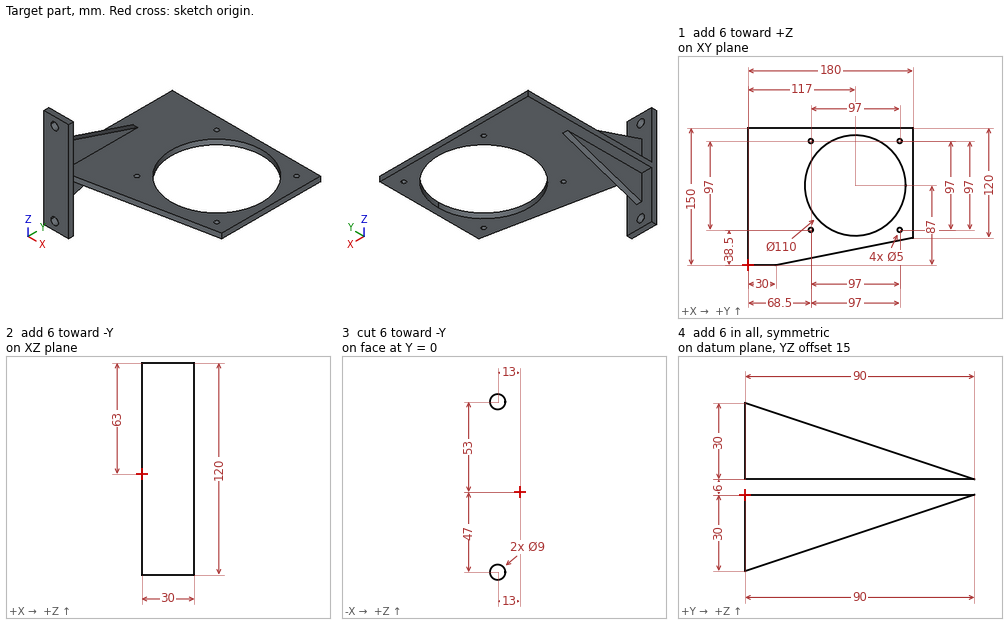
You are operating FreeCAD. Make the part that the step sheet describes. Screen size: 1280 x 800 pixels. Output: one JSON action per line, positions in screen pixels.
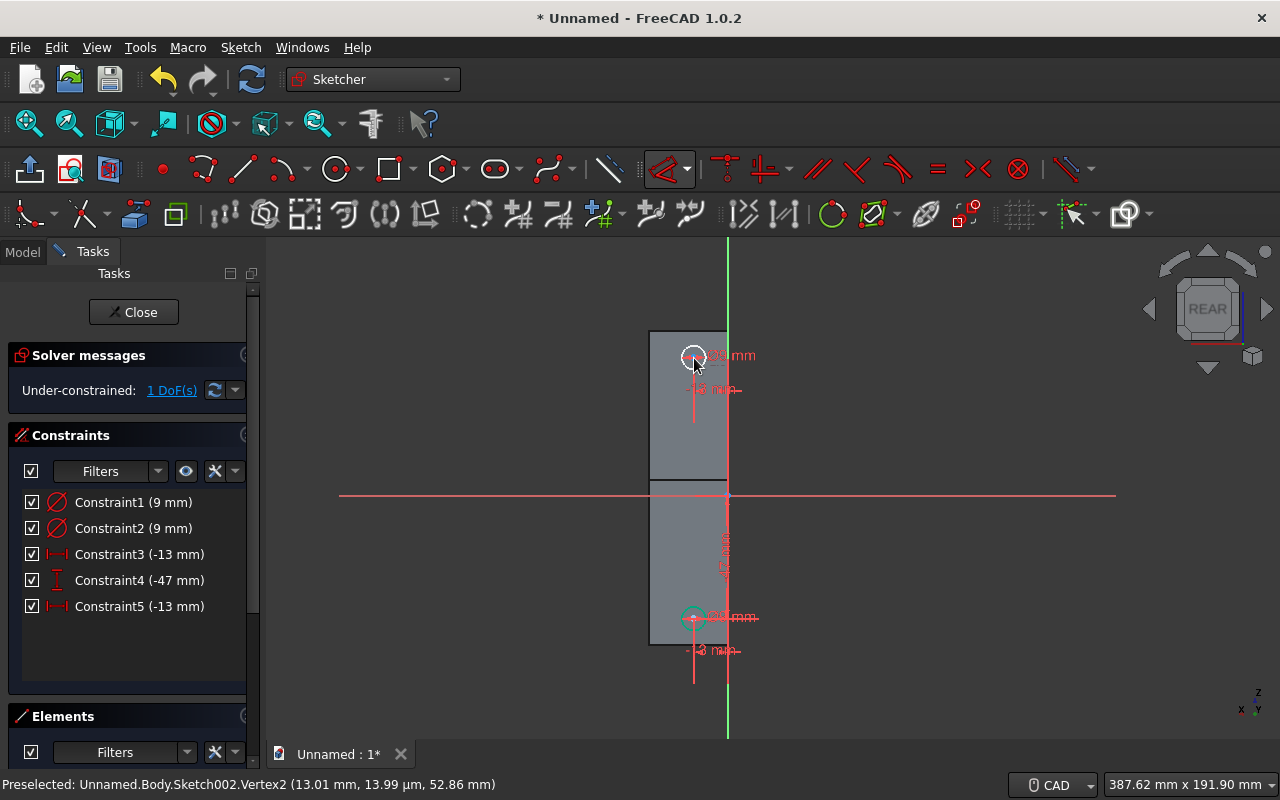
{"action": "left_click", "coordinate": [694, 358]}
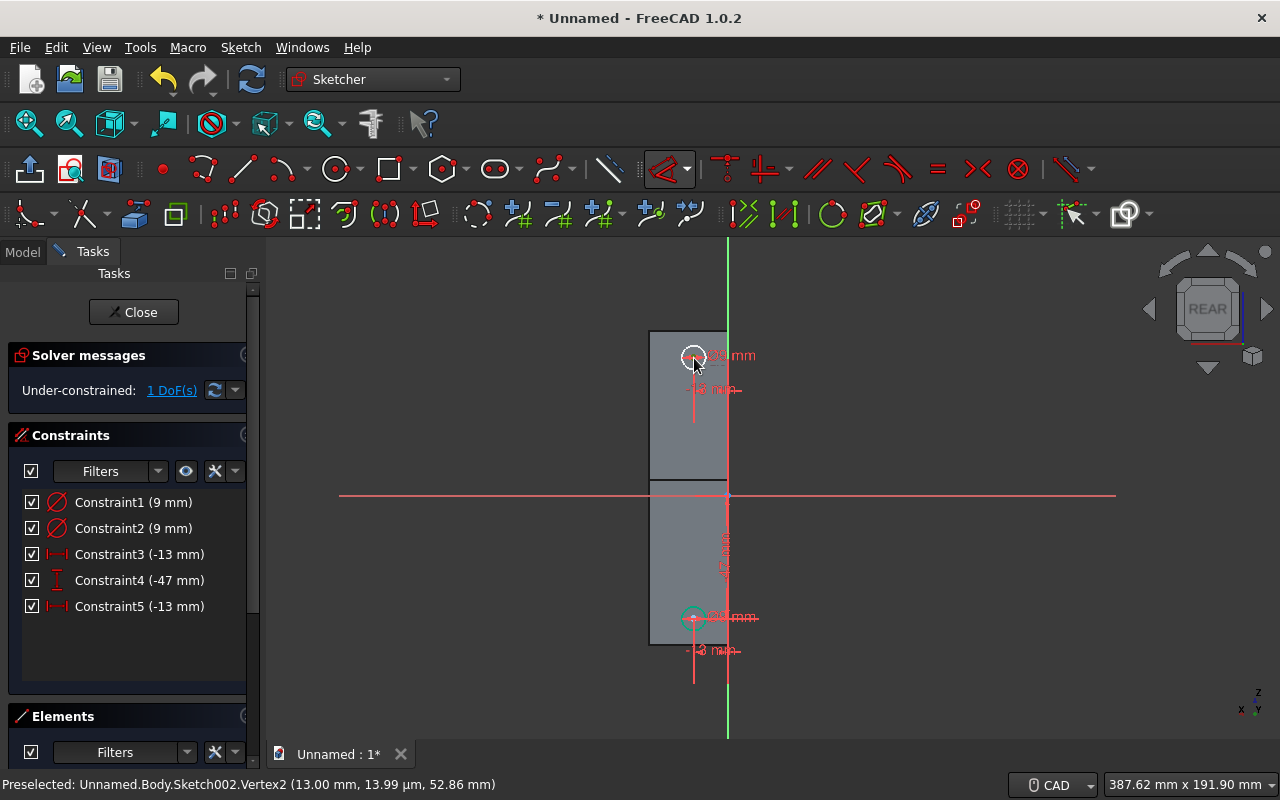
{"action": "key", "text": "i"}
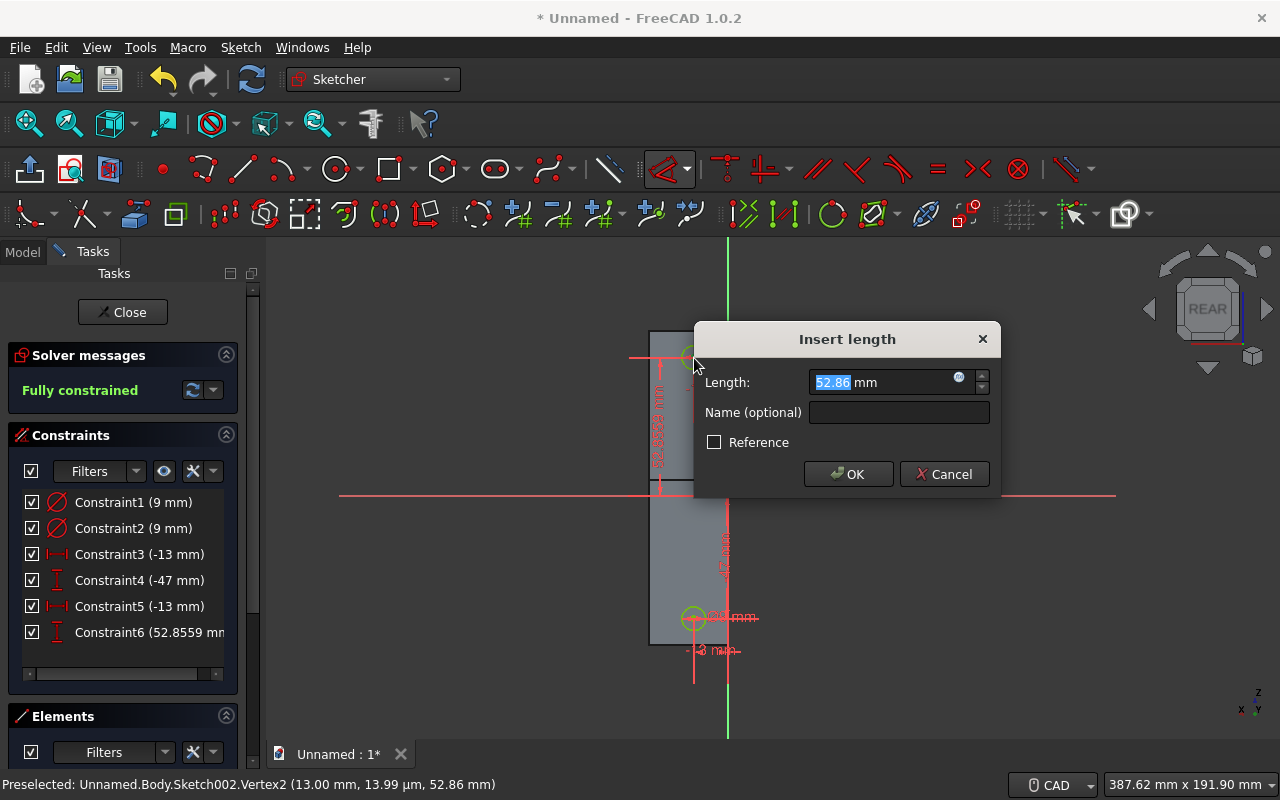
{"action": "type", "text": "53"}
{"action": "key", "text": "Return"}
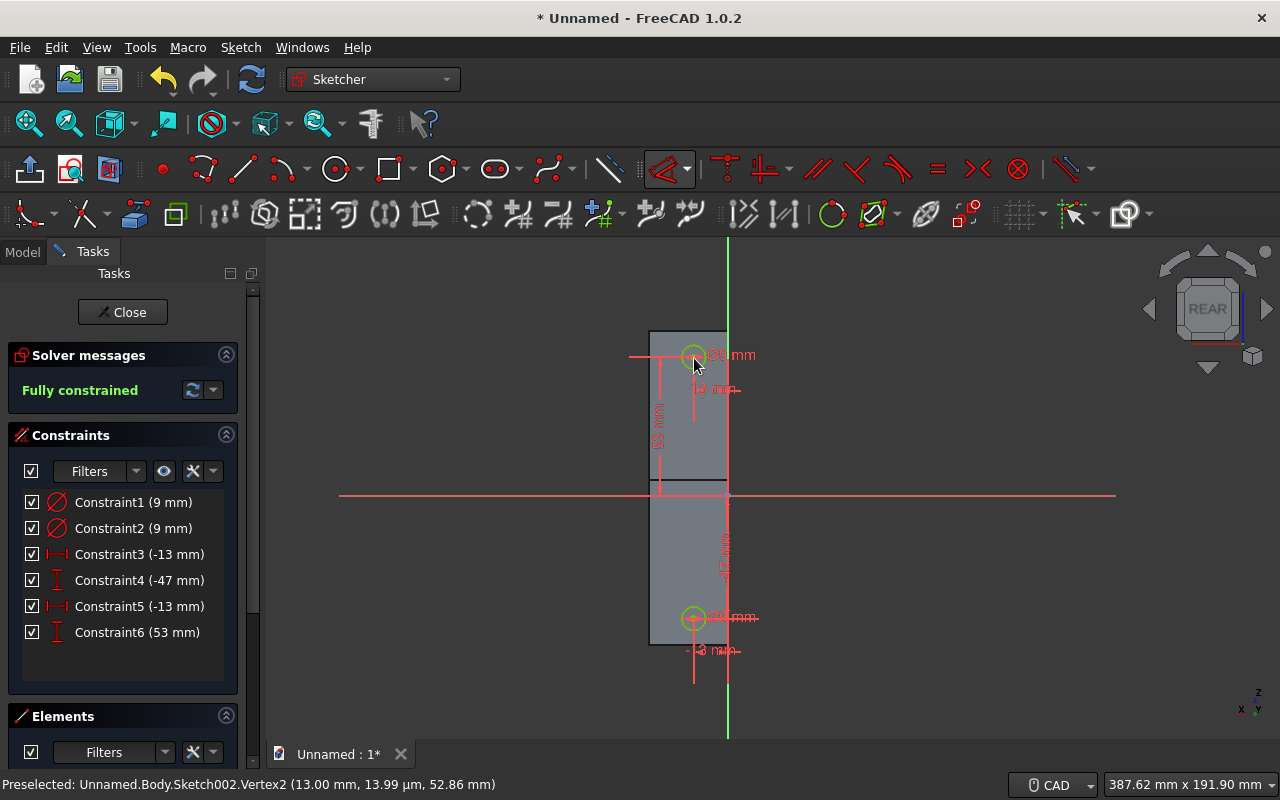
{"action": "left_click", "coordinate": [123, 312]}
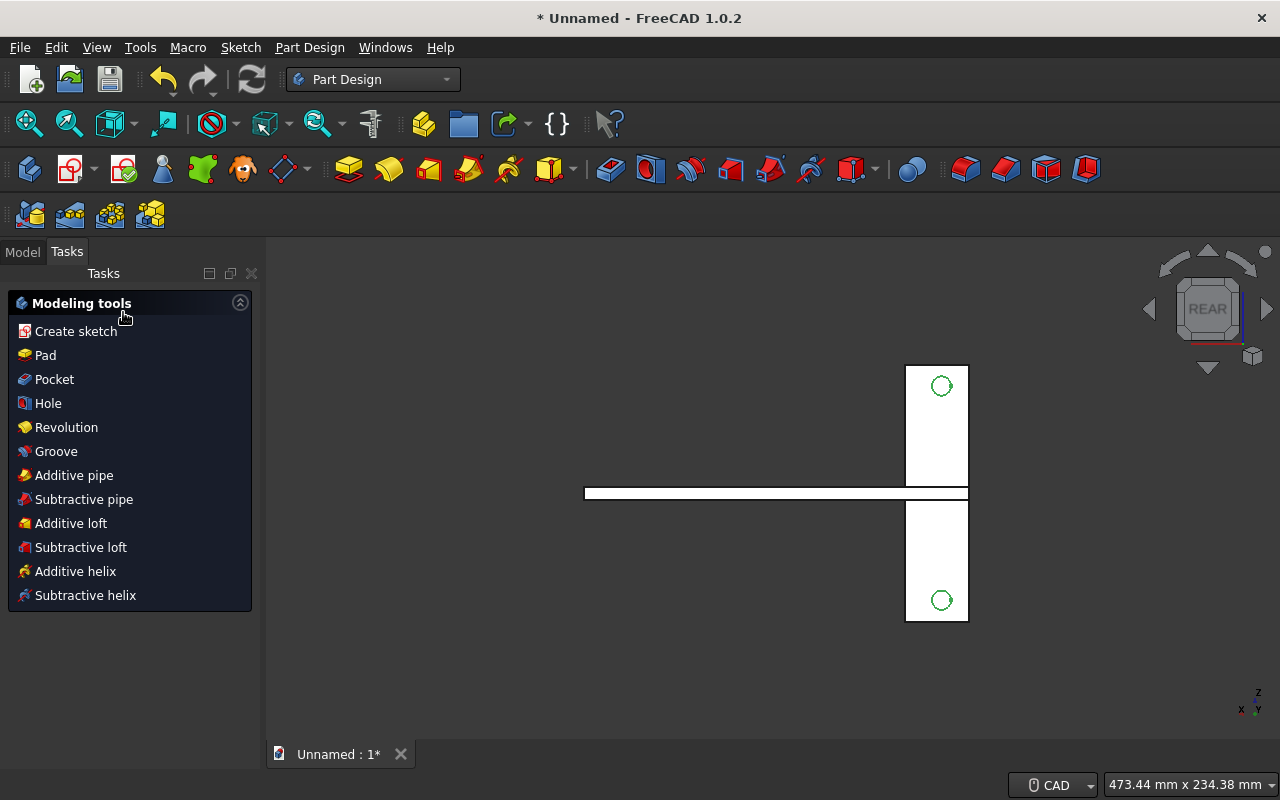
{"action": "left_click", "coordinate": [612, 170]}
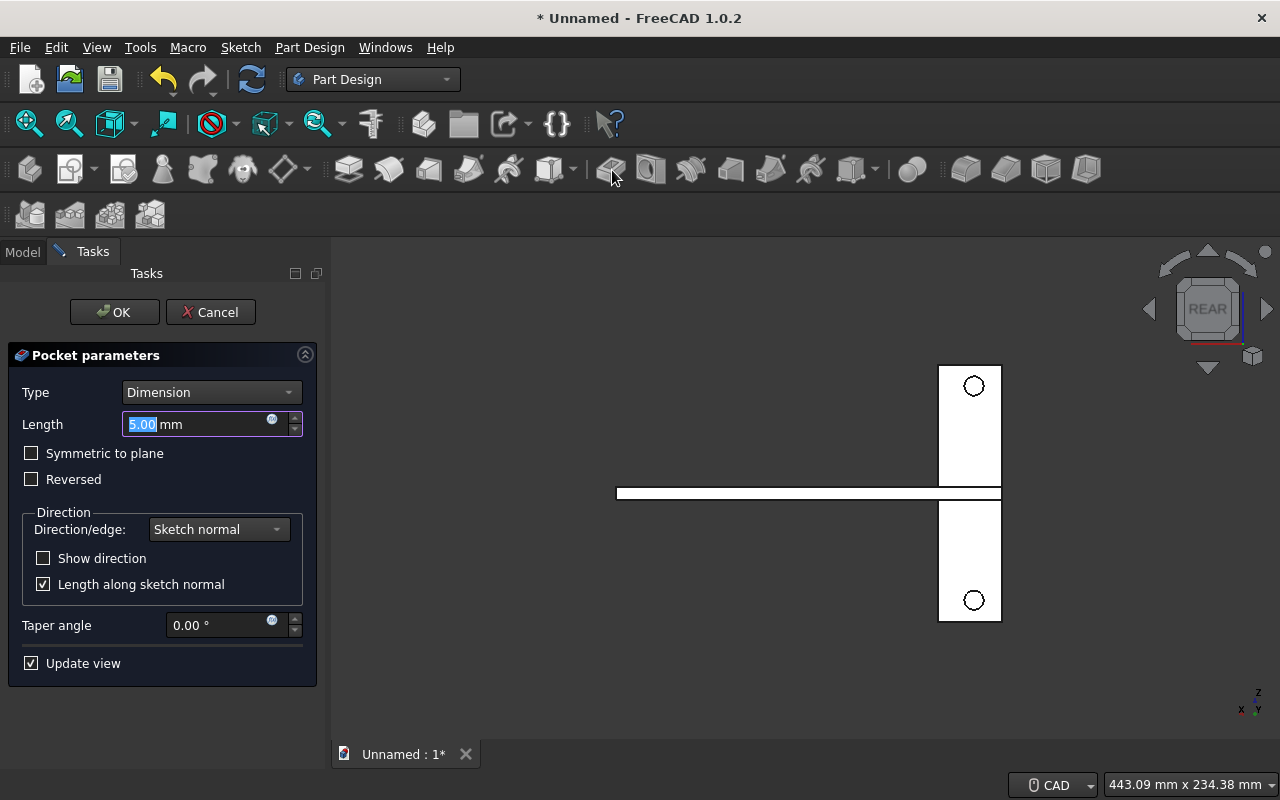
{"action": "type", "text": "6"}
{"action": "key", "text": "Tab"}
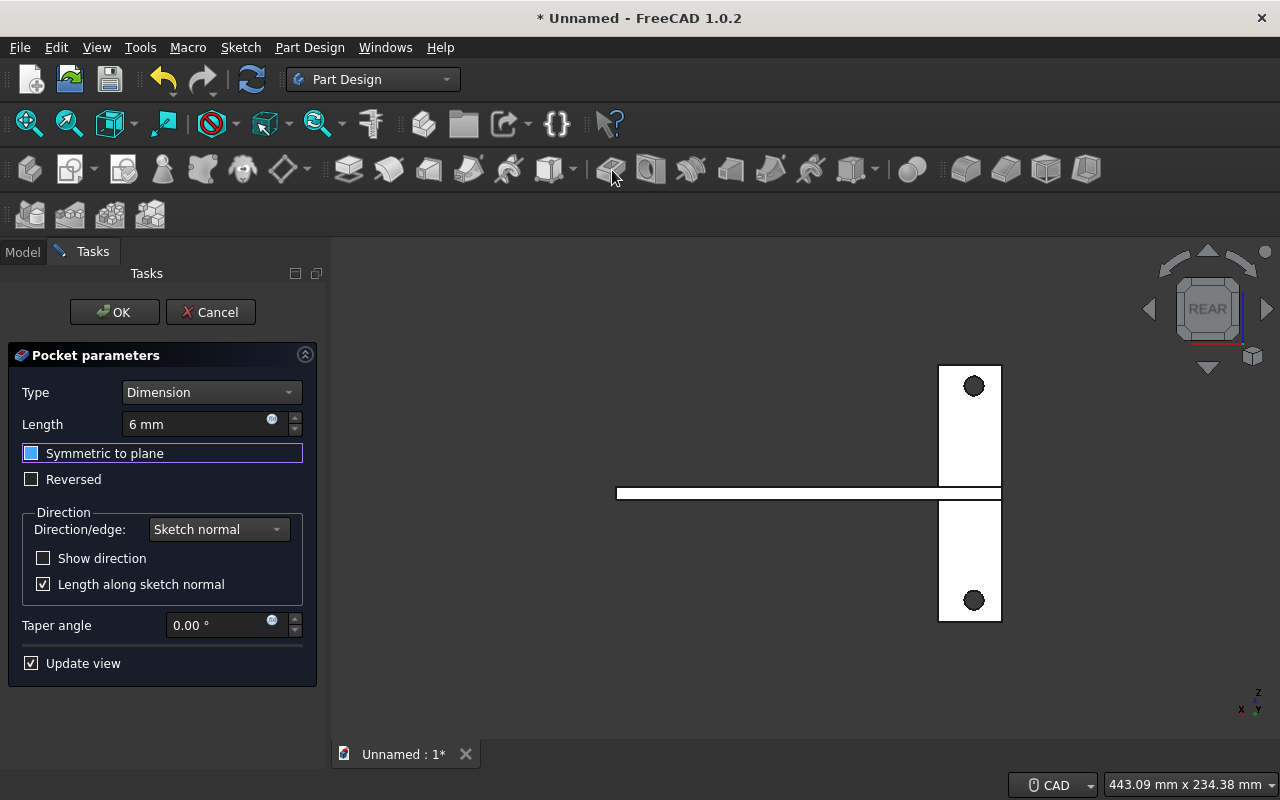
{"action": "left_click", "coordinate": [115, 312]}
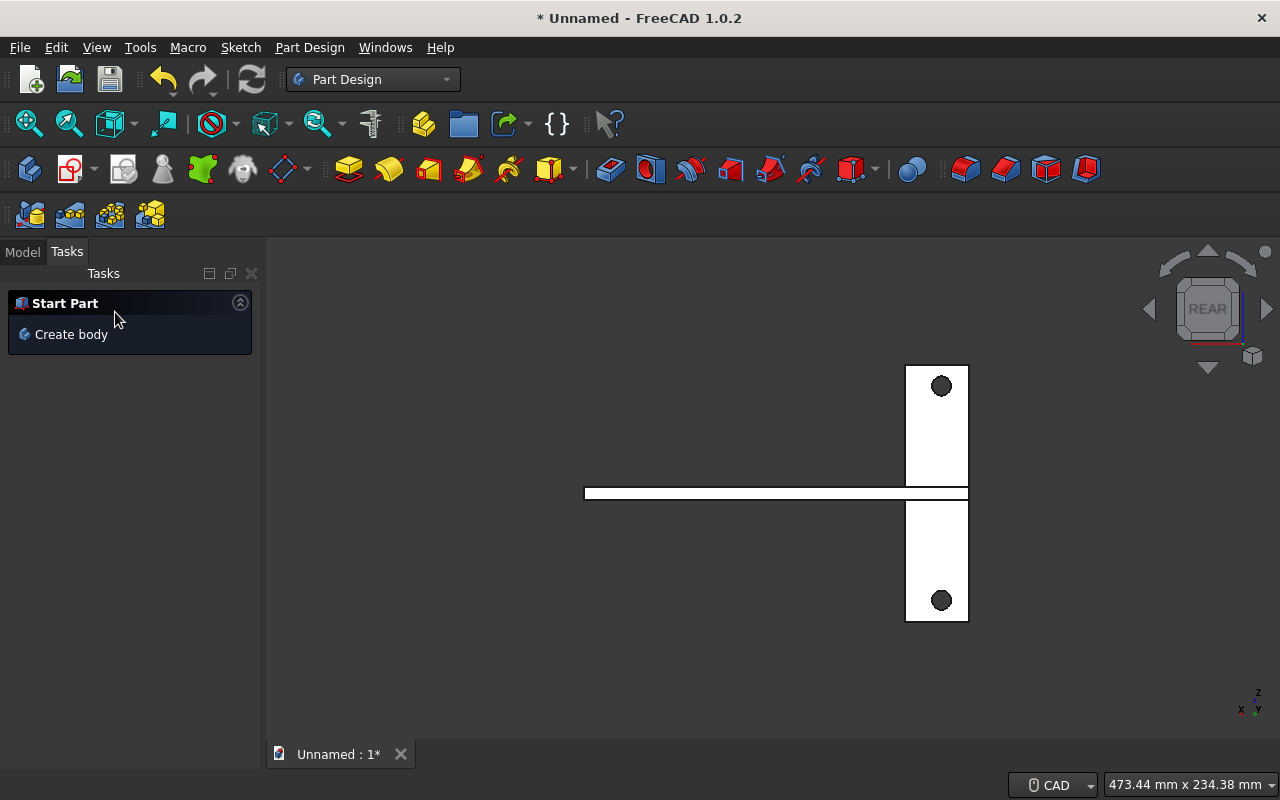
{"action": "left_click", "coordinate": [23, 251]}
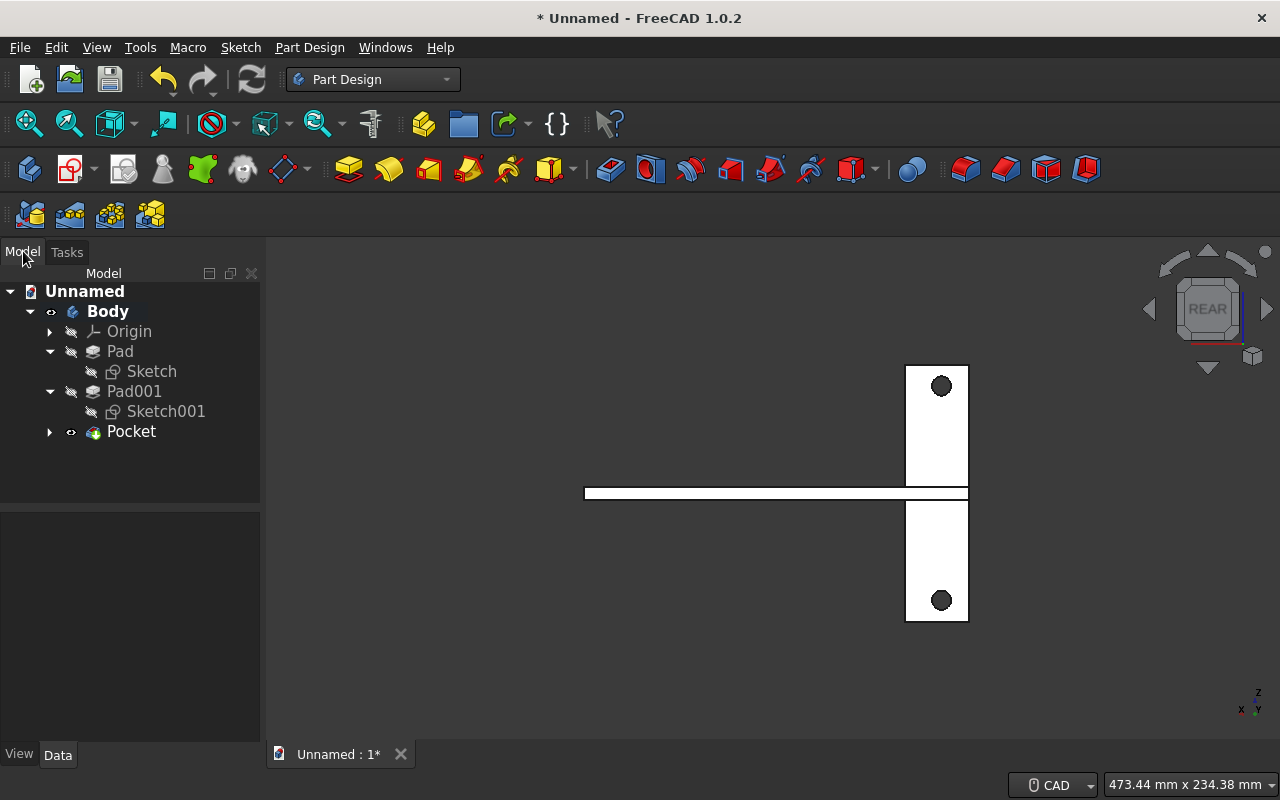
{"action": "left_click", "coordinate": [50, 332]}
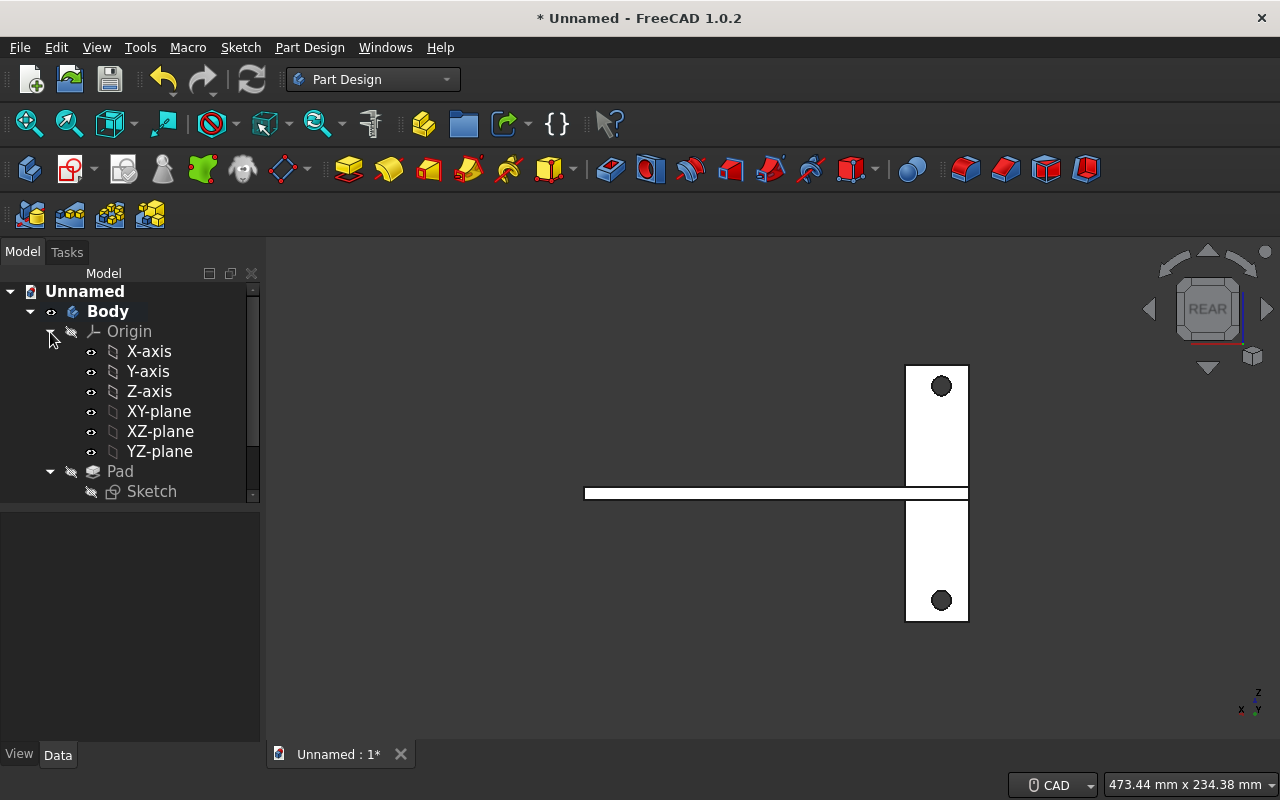
{"action": "left_click", "coordinate": [136, 452]}